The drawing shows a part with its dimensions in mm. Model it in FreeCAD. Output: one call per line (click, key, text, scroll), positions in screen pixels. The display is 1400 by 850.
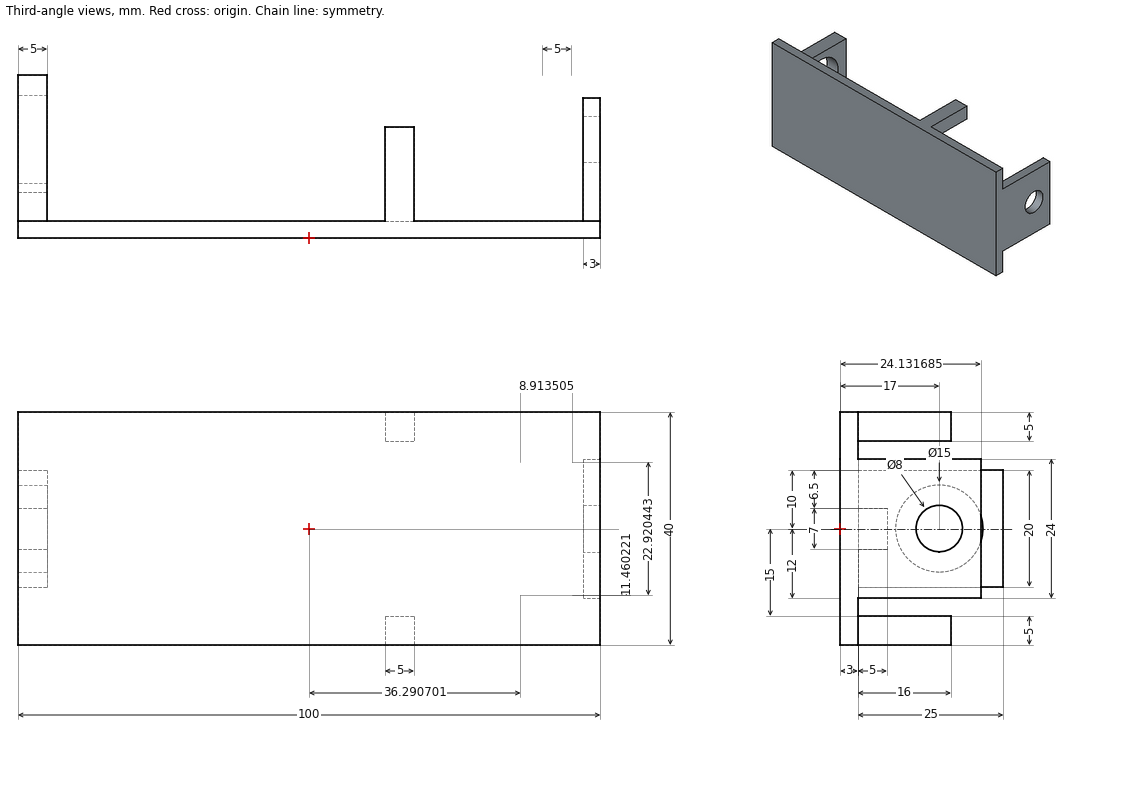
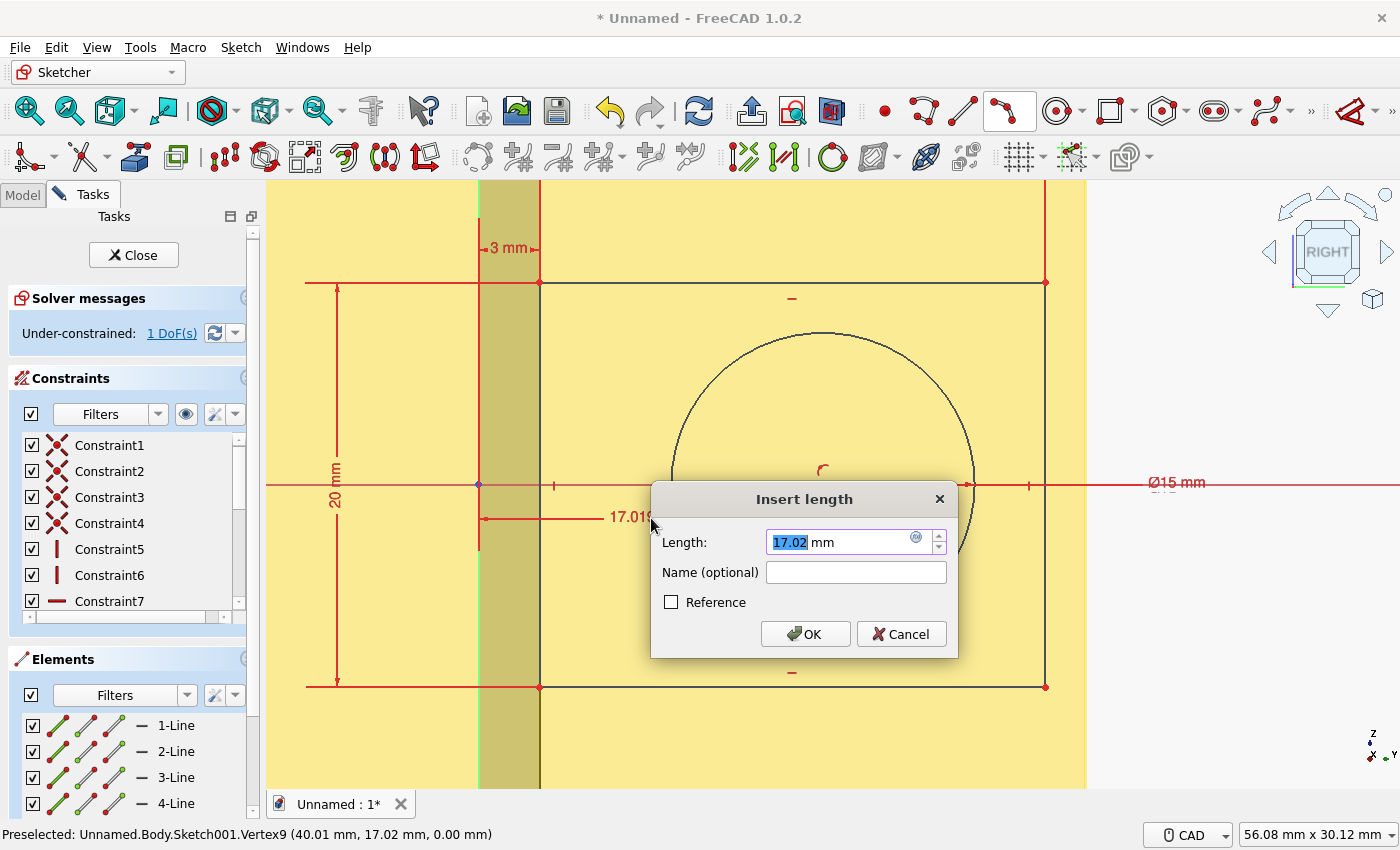
text(17)
key(Return)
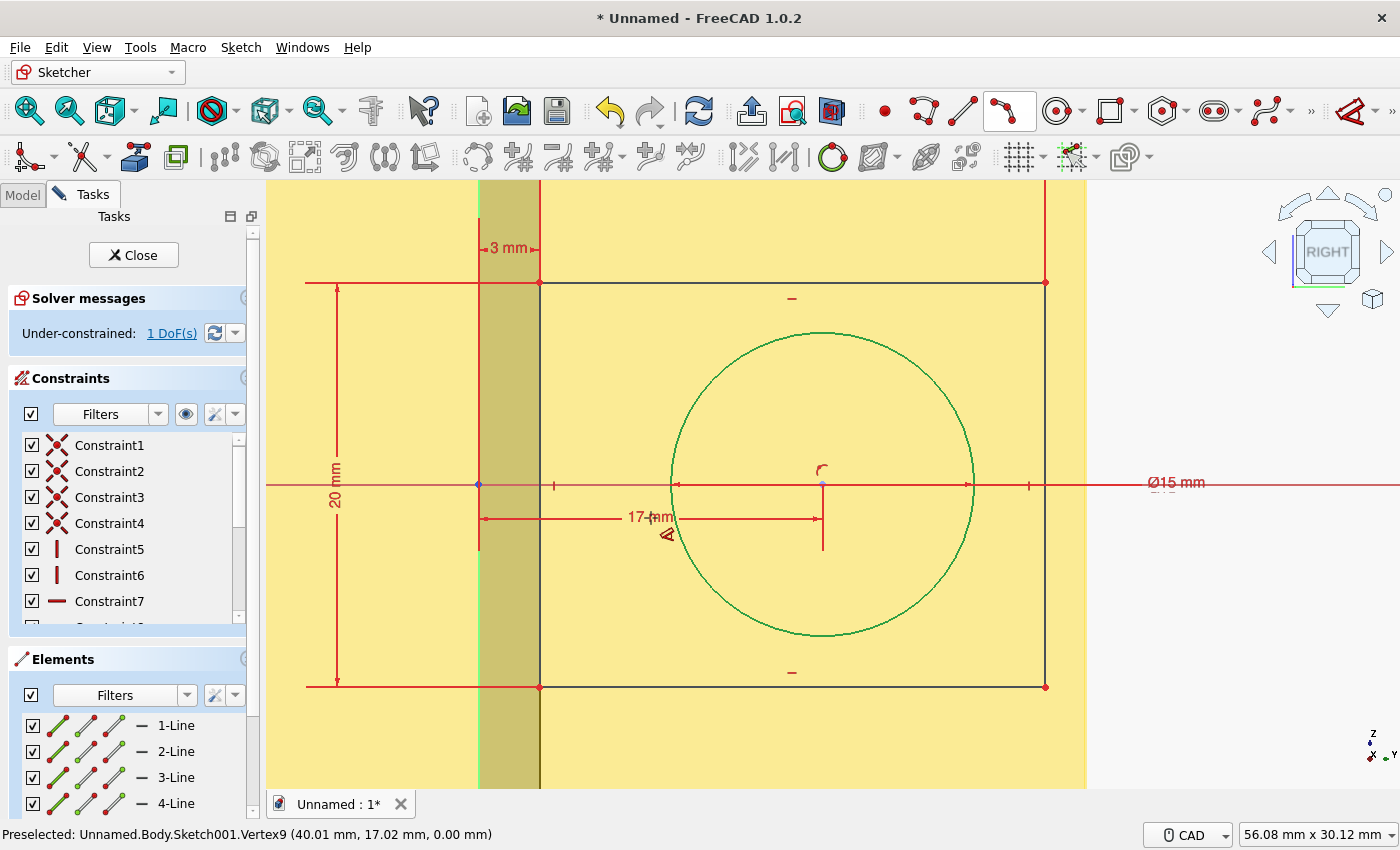
click(540, 283)
click(445, 384)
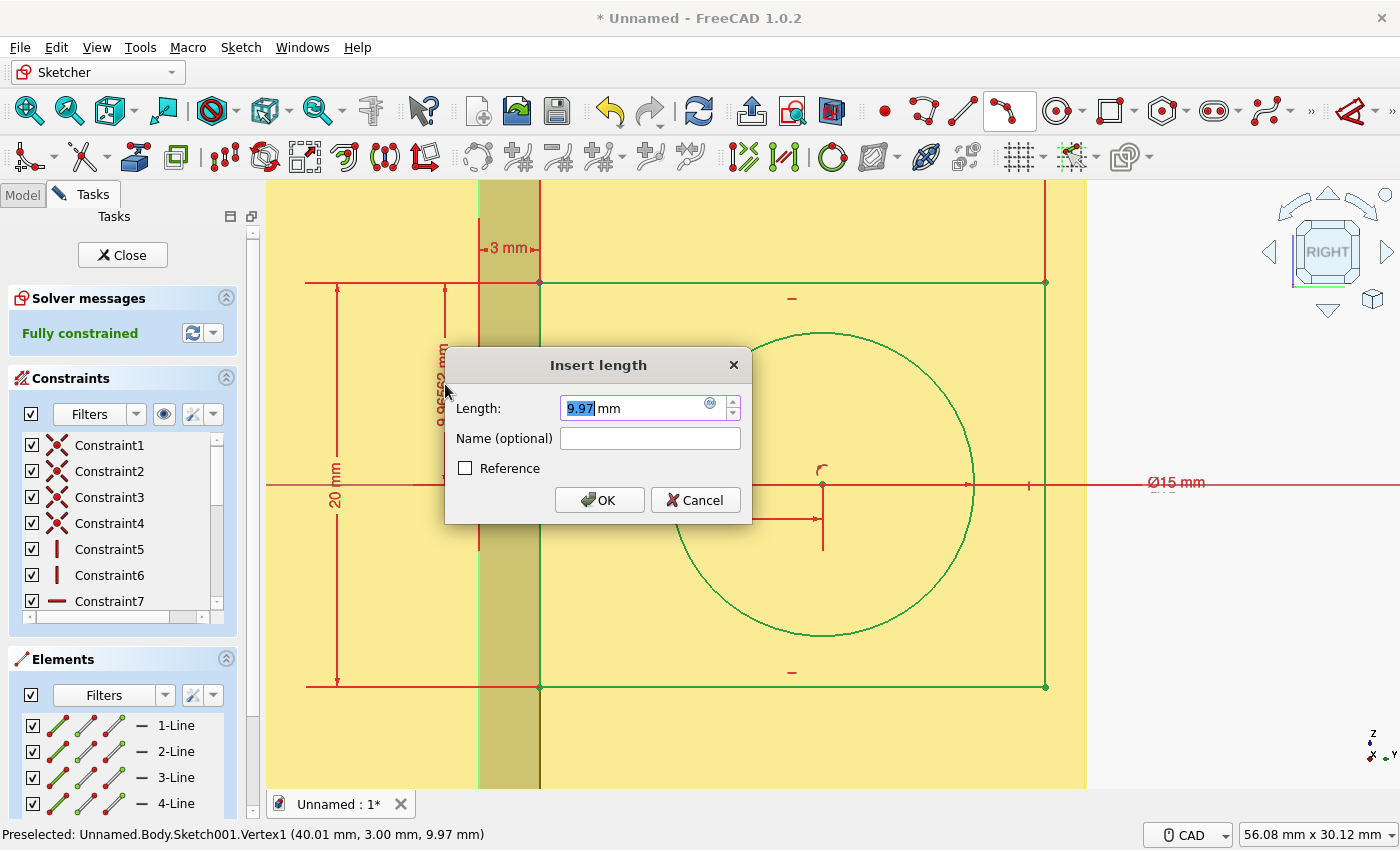
text(10)
key(Return)
key(Escape)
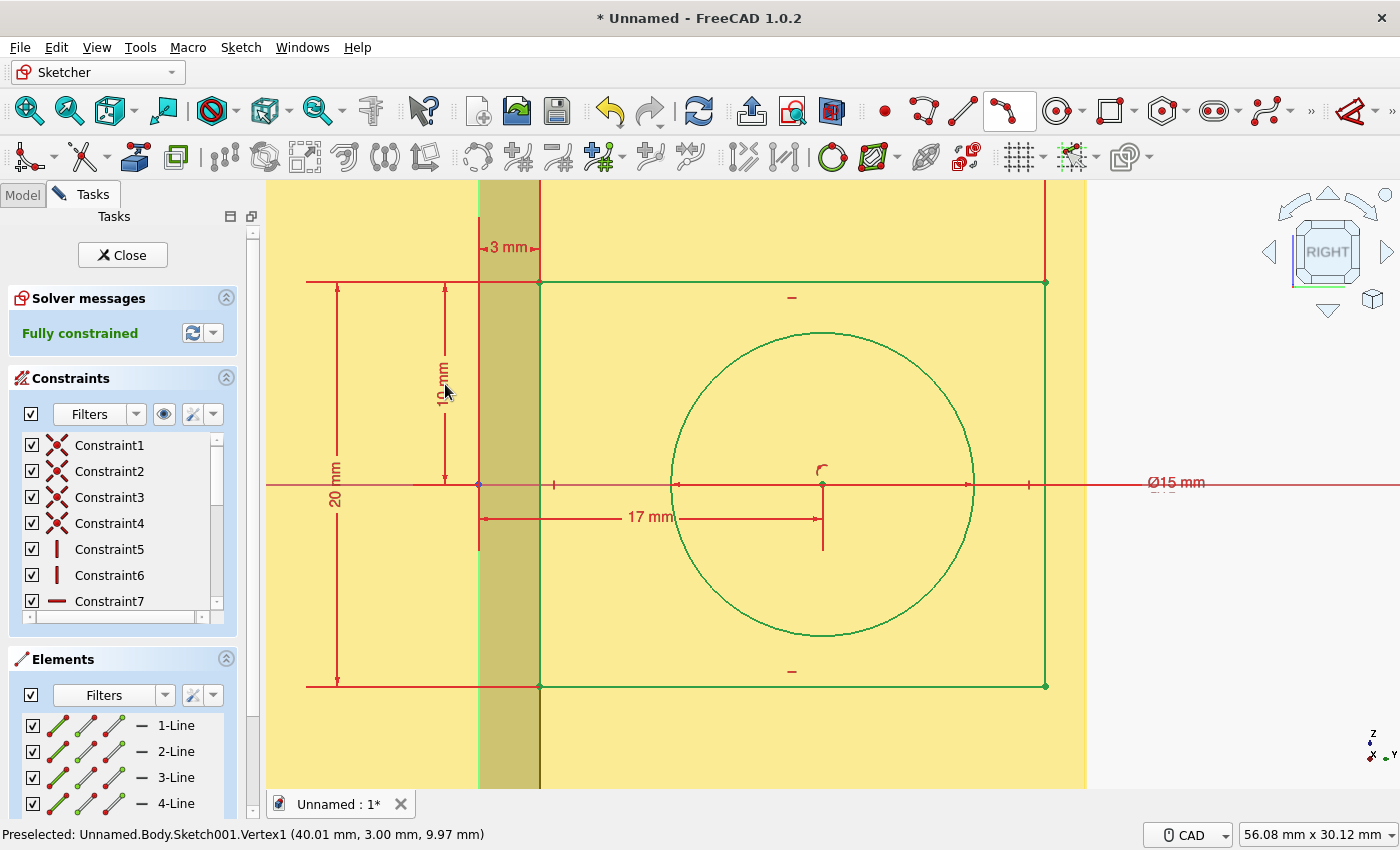
click(123, 255)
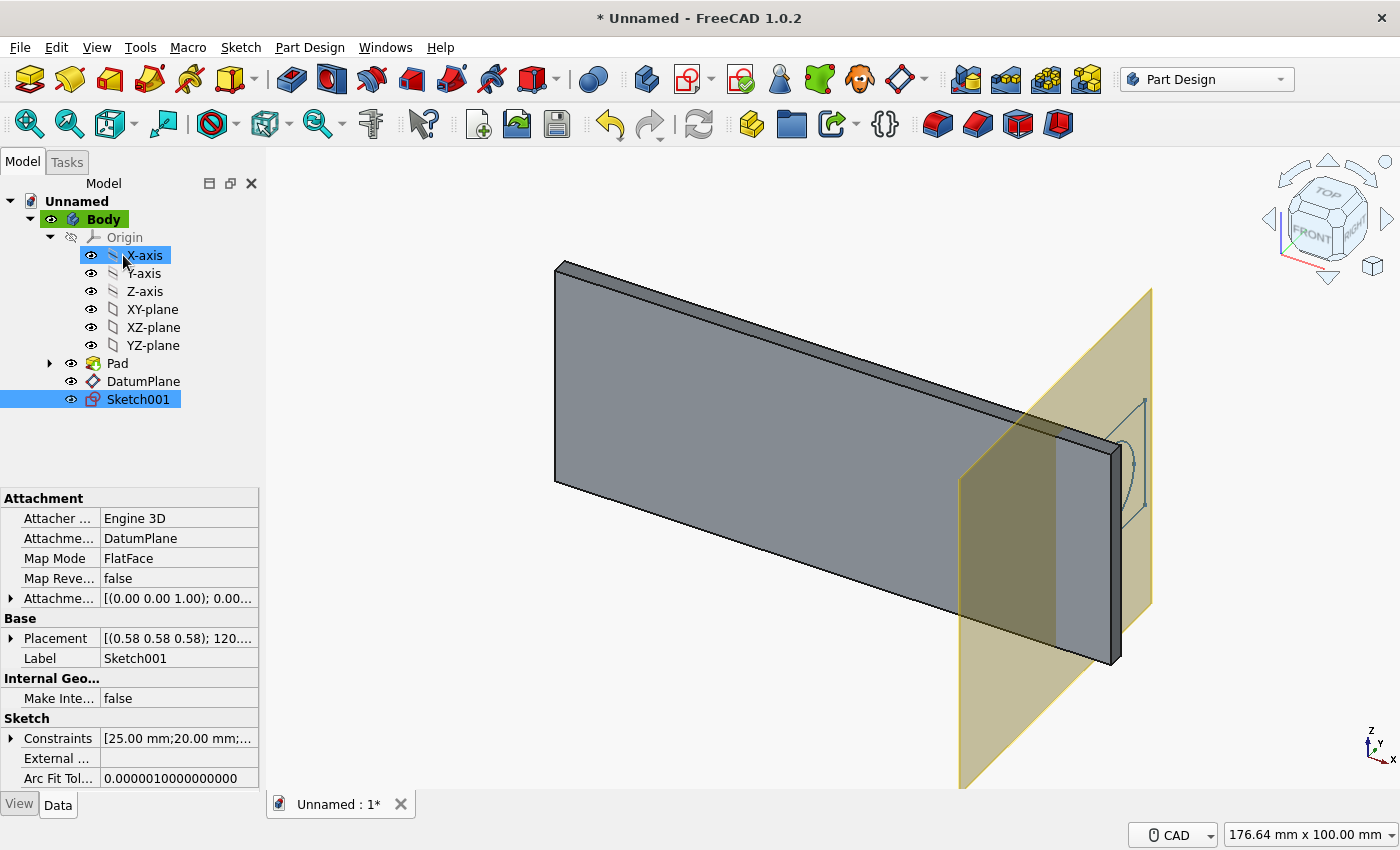
click(30, 80)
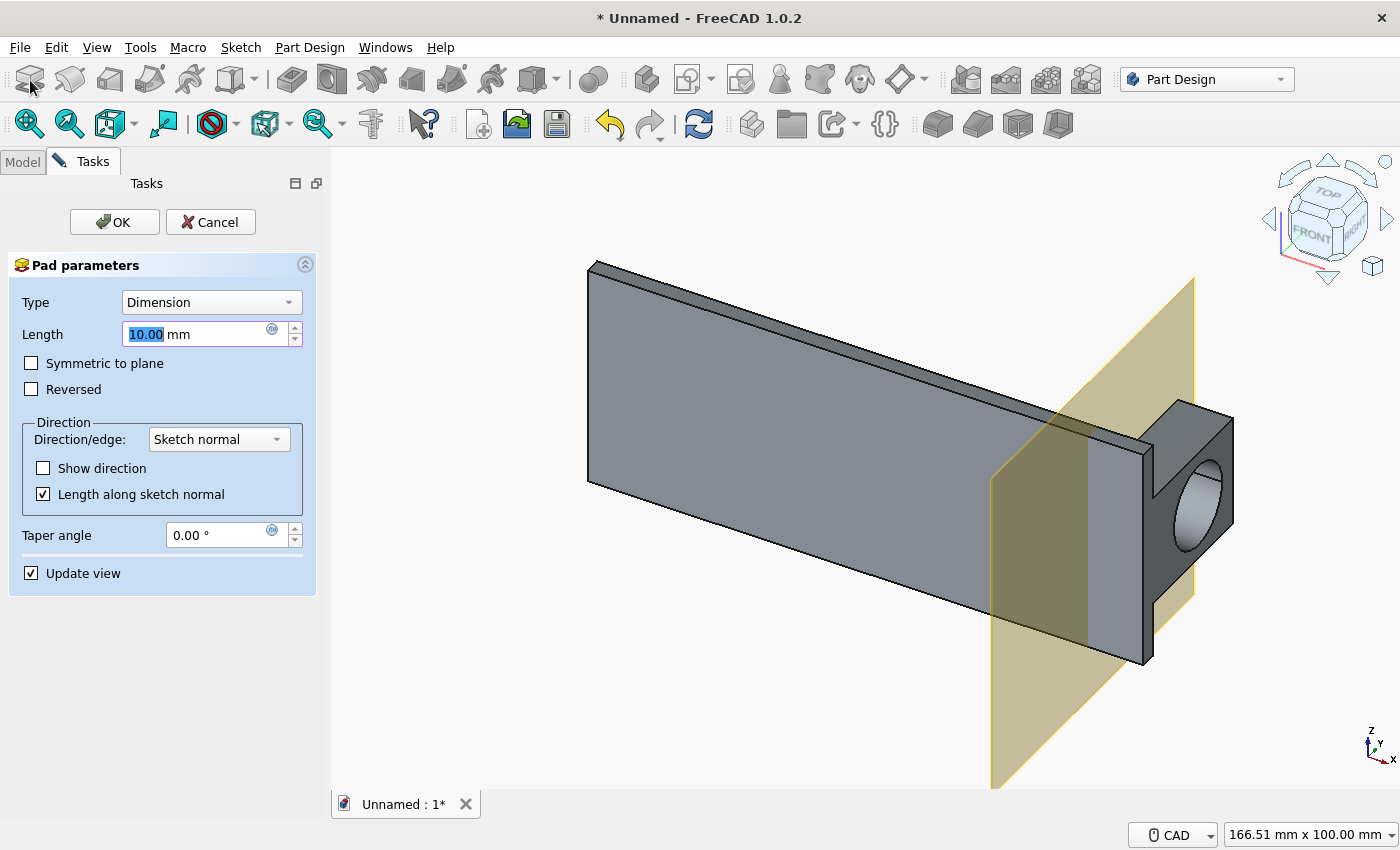
text(5)
key(Tab)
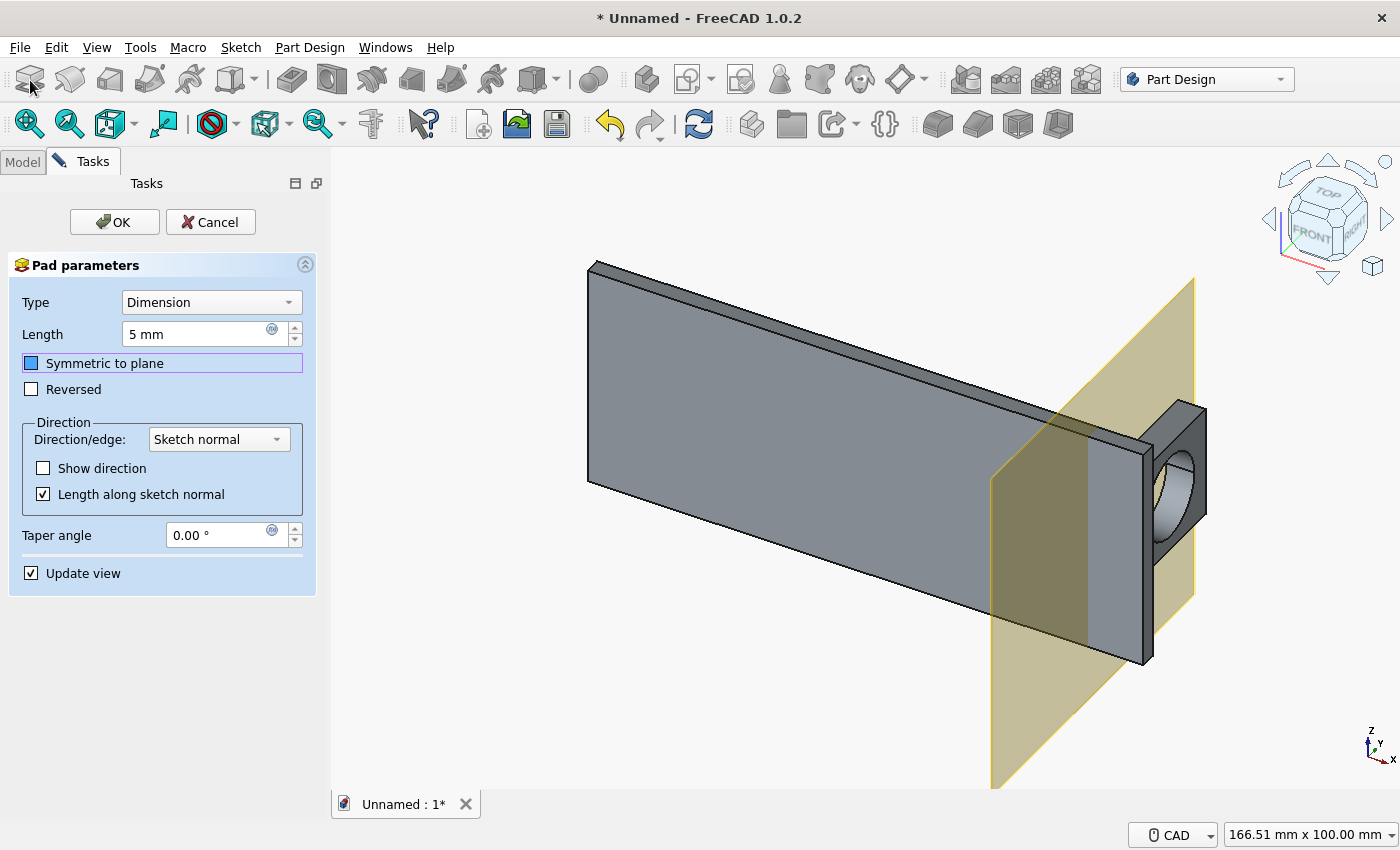
click(115, 222)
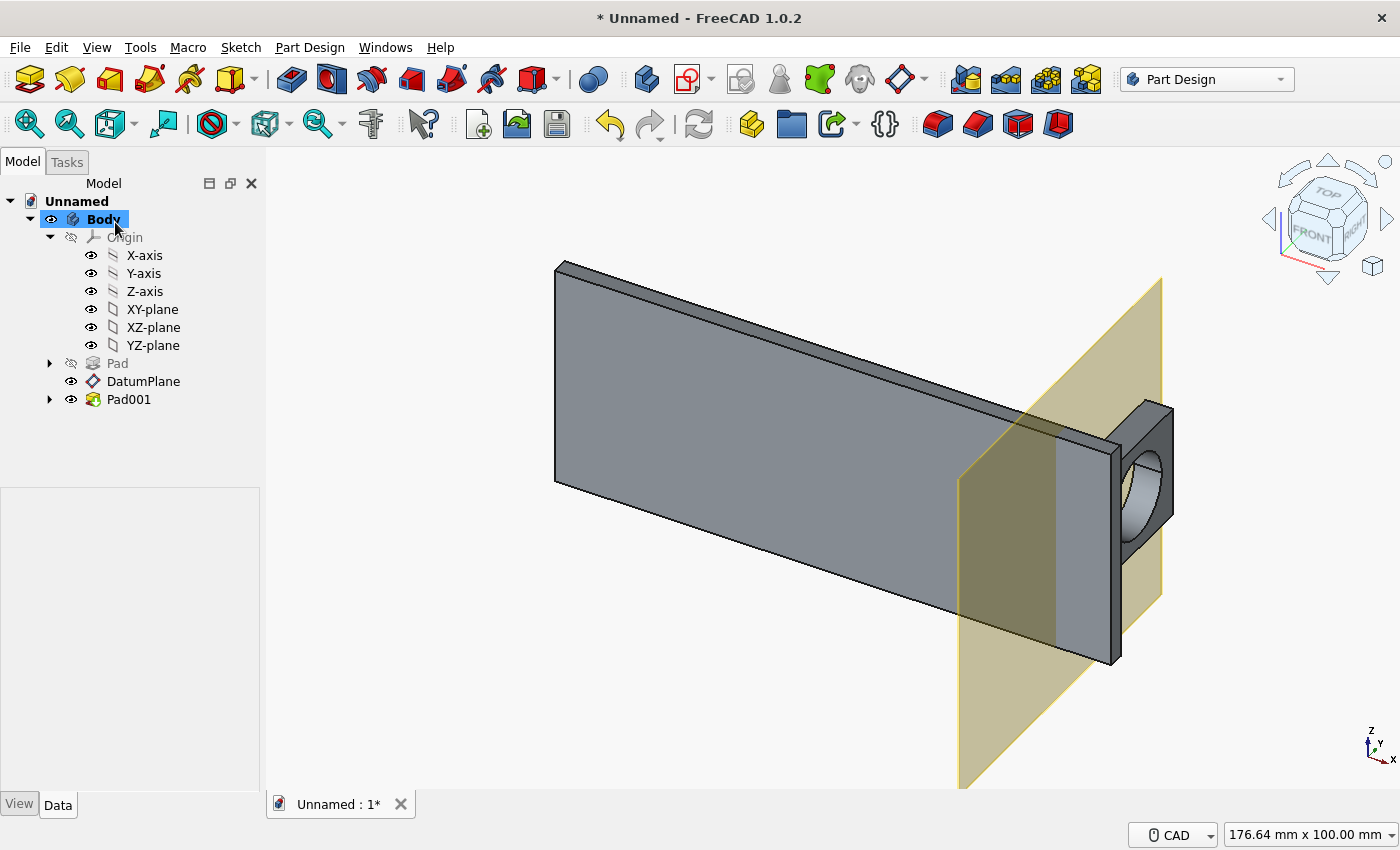
click(116, 381)
key(space)